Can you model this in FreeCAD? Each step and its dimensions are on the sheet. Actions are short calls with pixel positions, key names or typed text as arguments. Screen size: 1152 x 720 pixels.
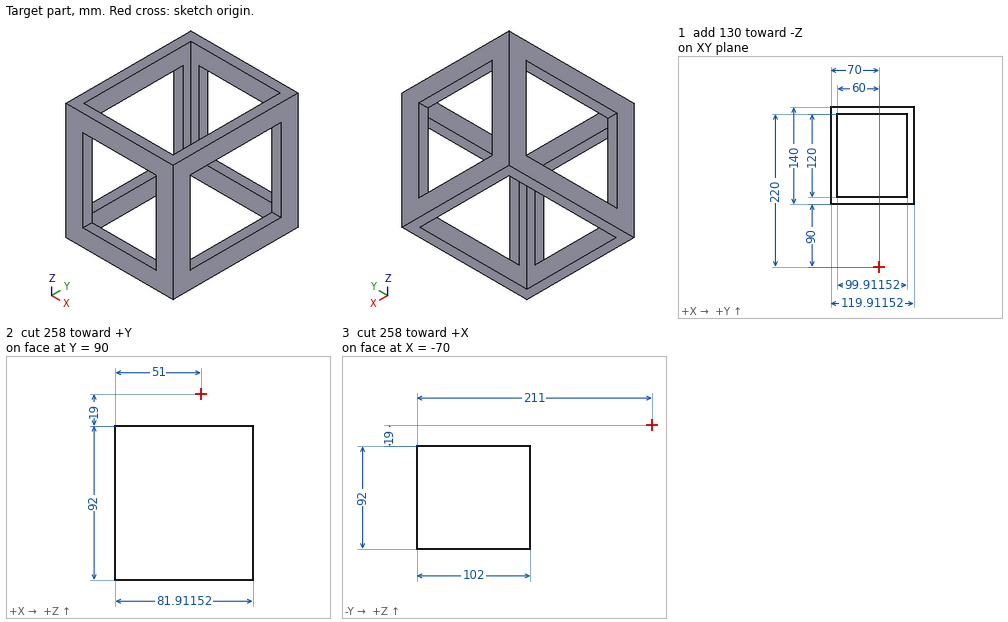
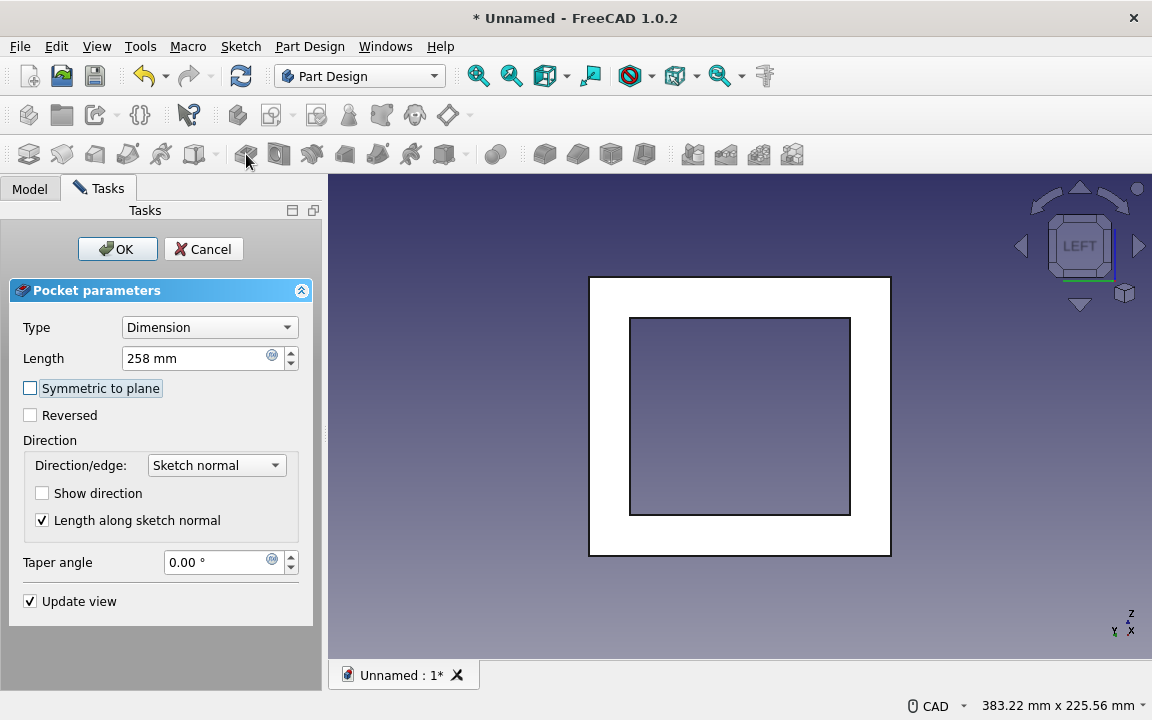
click(118, 249)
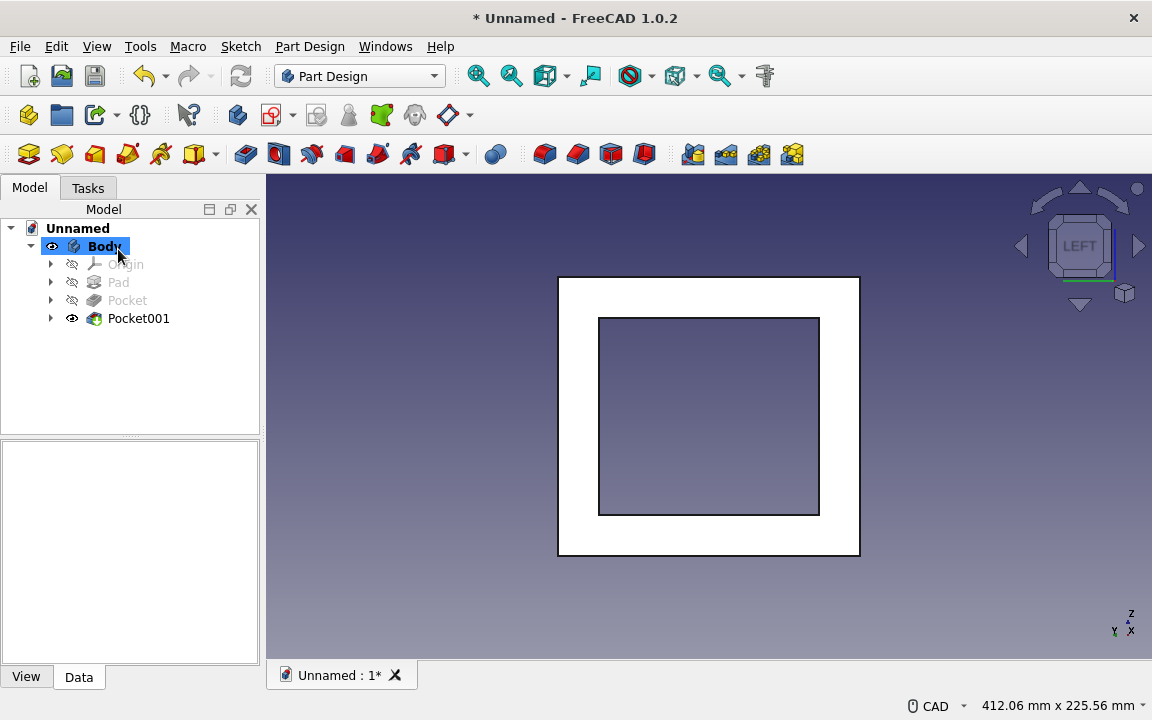
key(0)